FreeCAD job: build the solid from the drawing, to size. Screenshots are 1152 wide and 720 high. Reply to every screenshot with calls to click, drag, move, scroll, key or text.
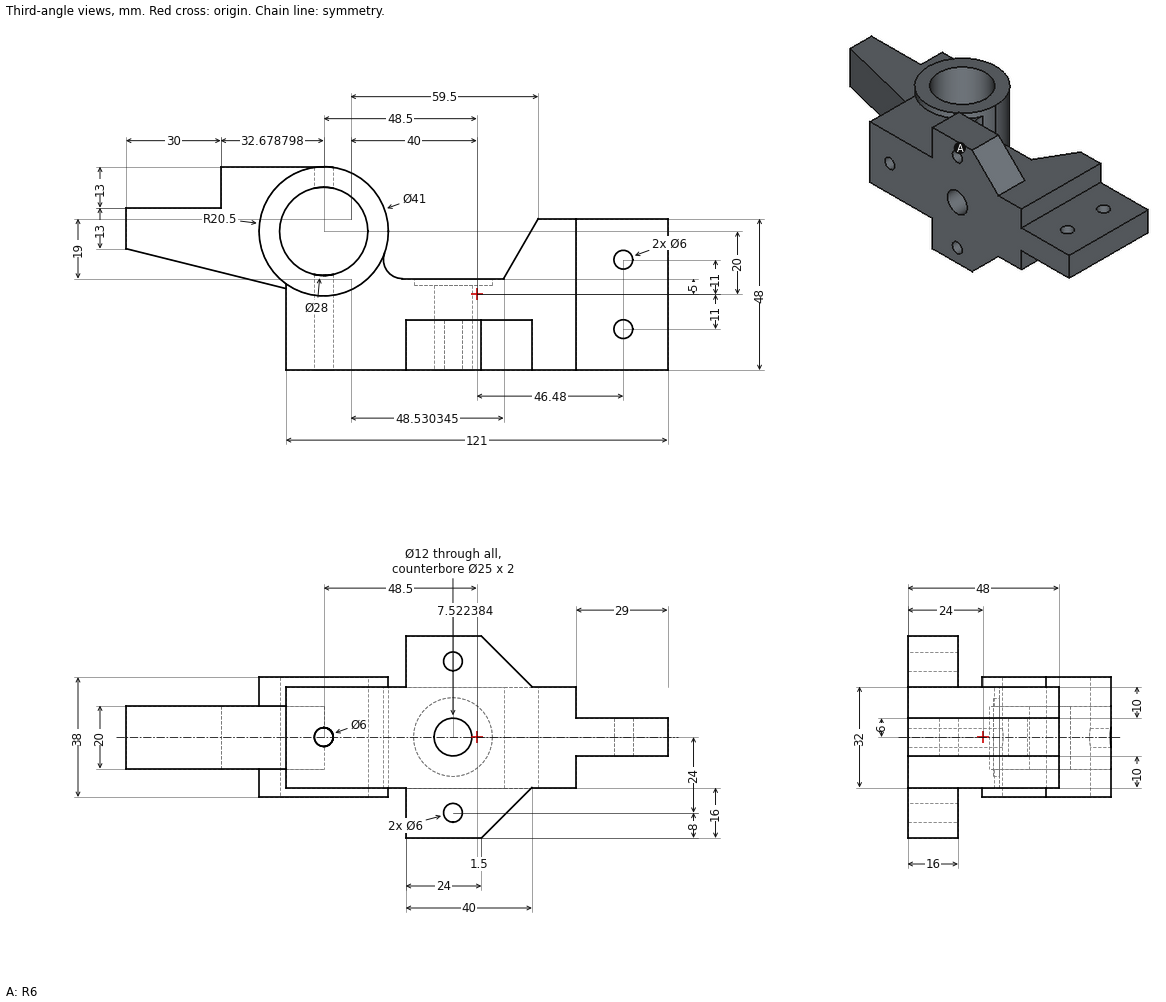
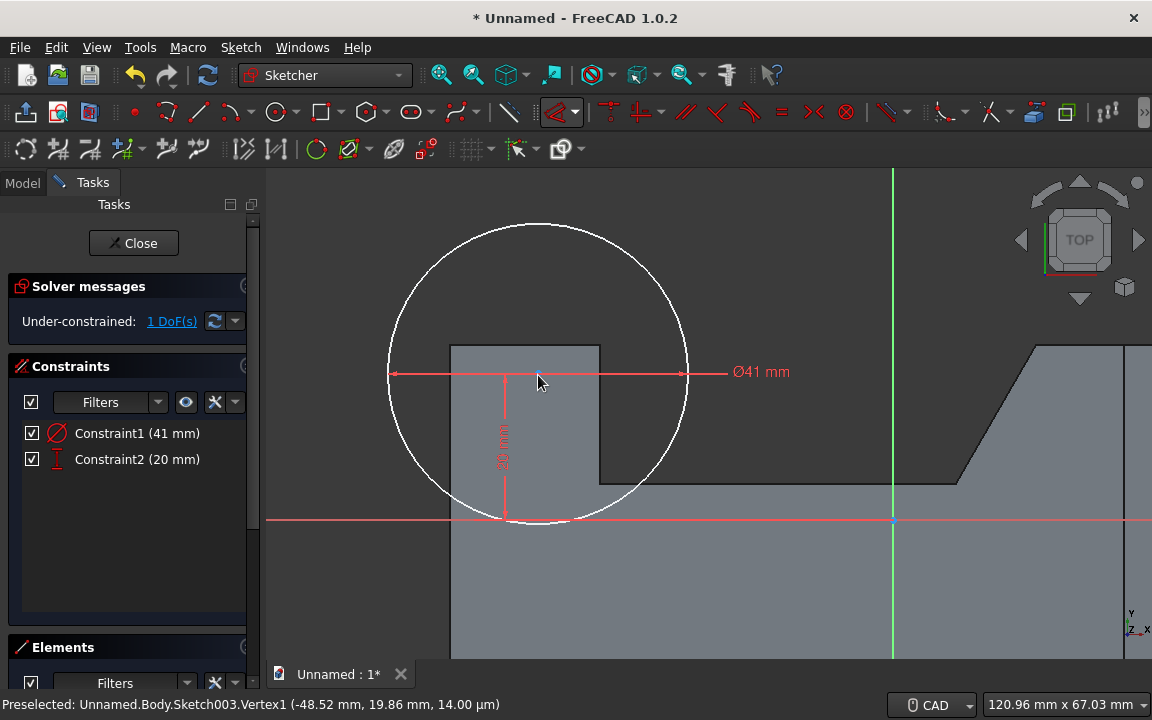
click(538, 374)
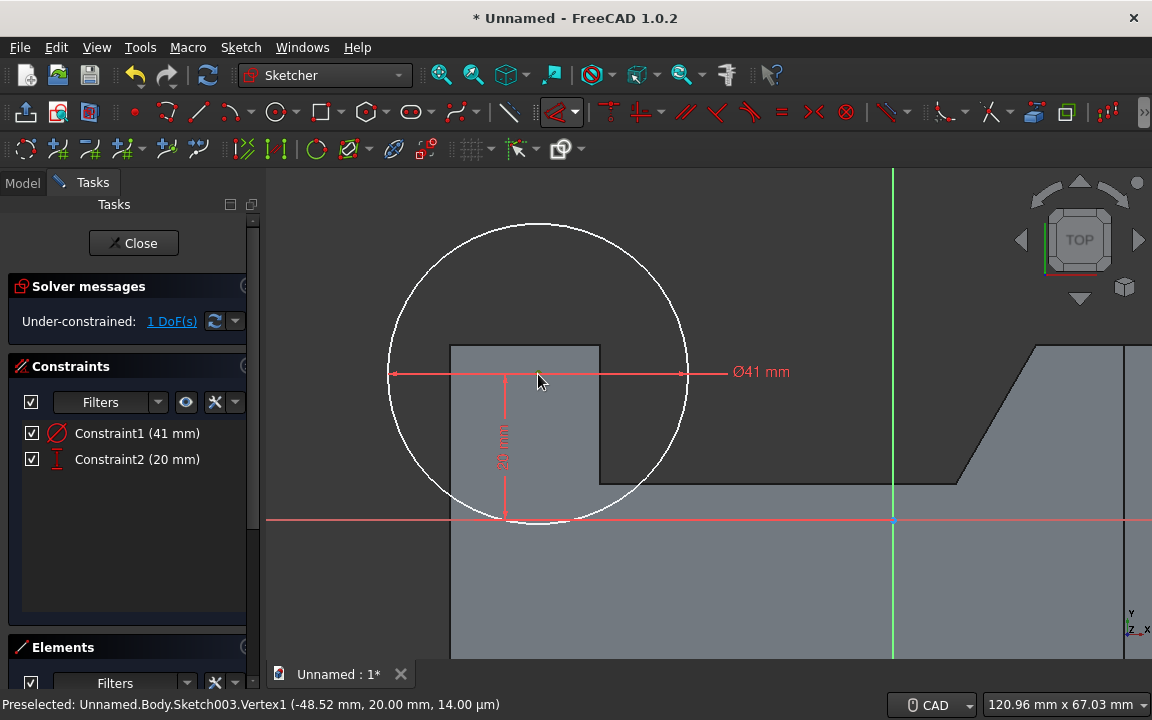
key(l)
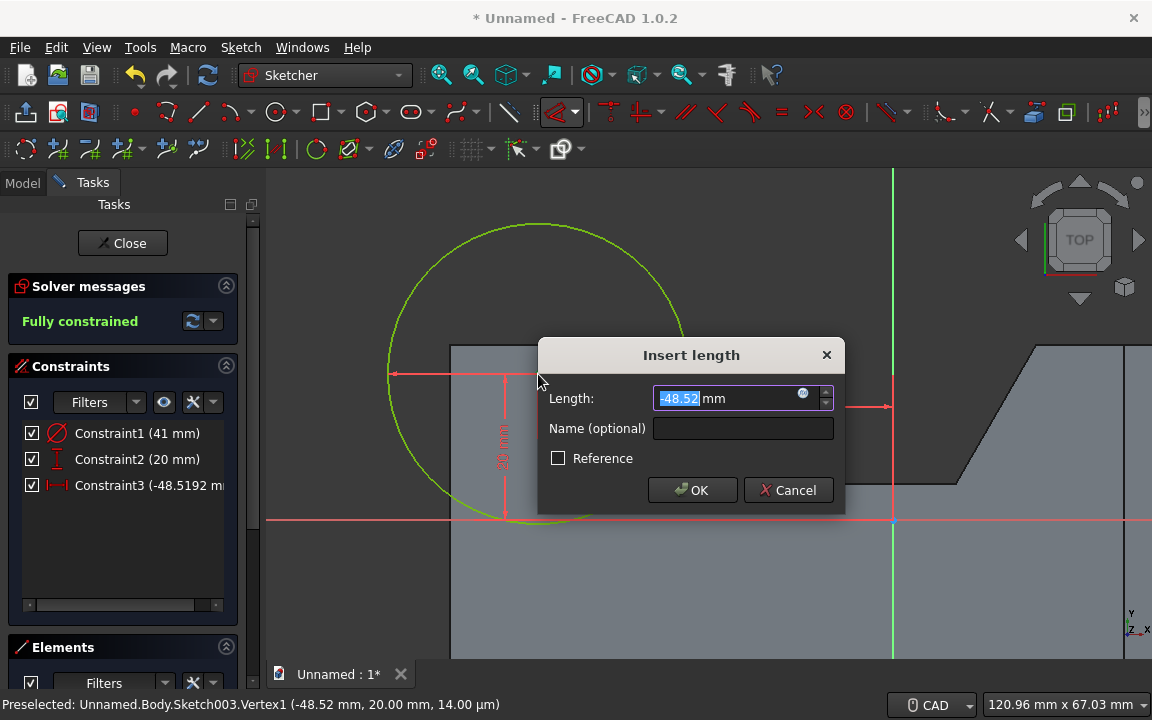
text(-48.5)
key(Return)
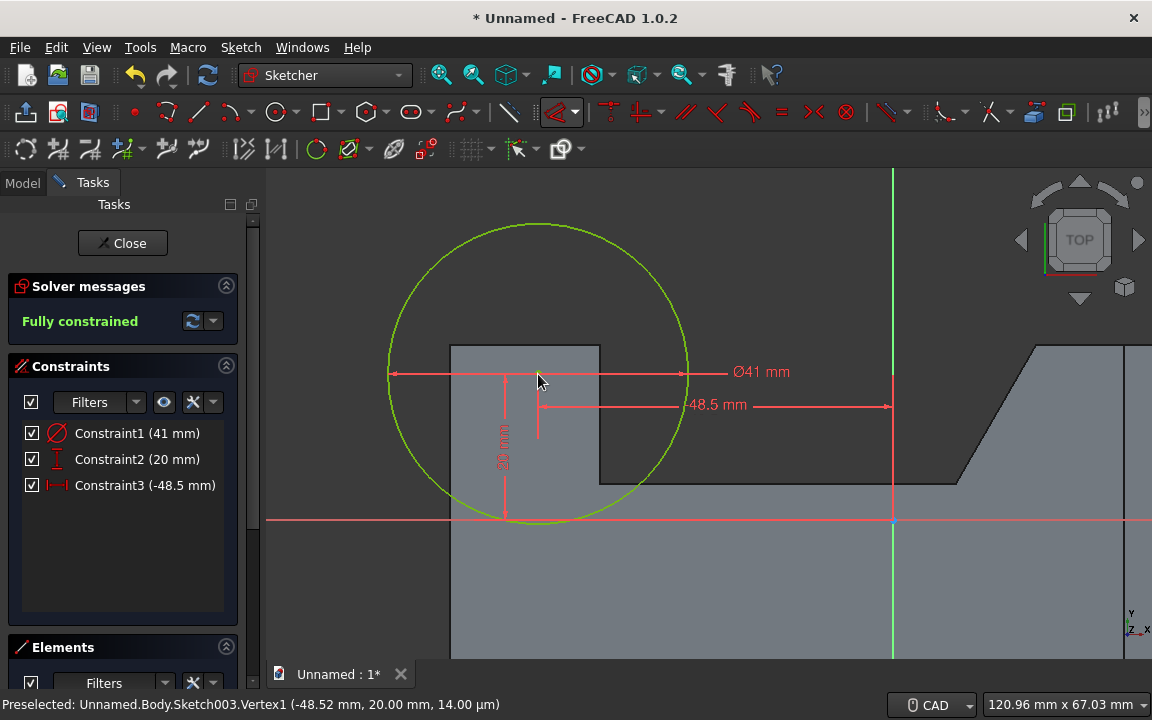
click(123, 243)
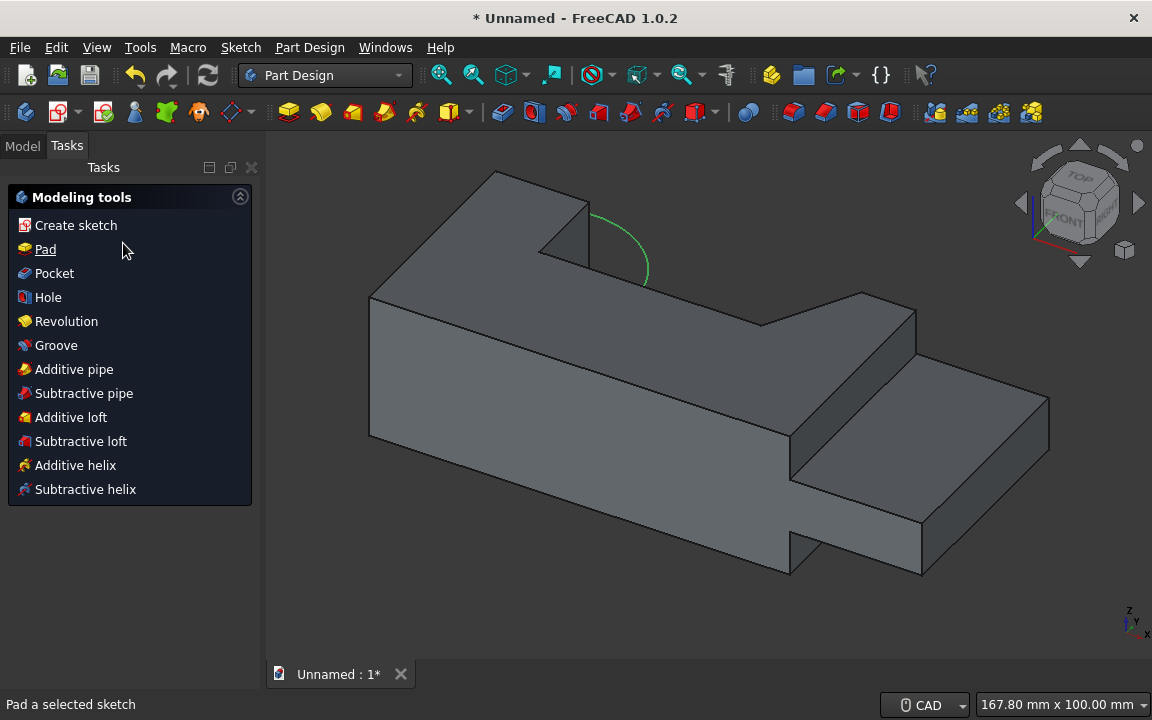
click(290, 112)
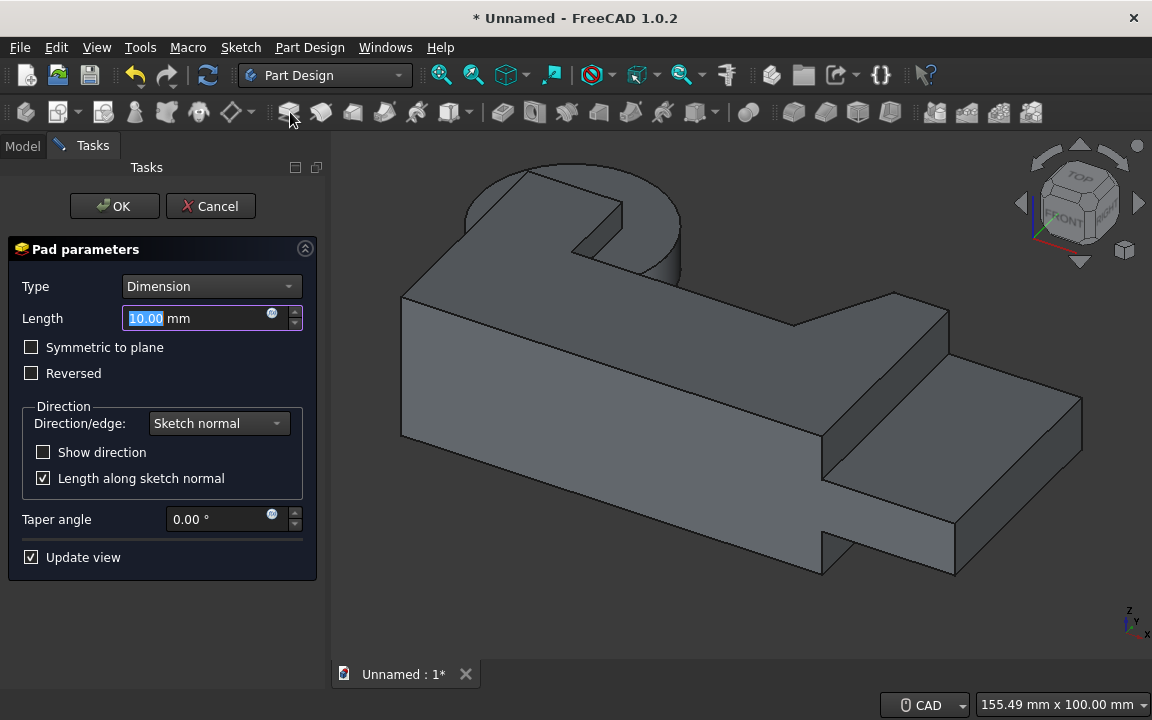
text(38)
key(Tab)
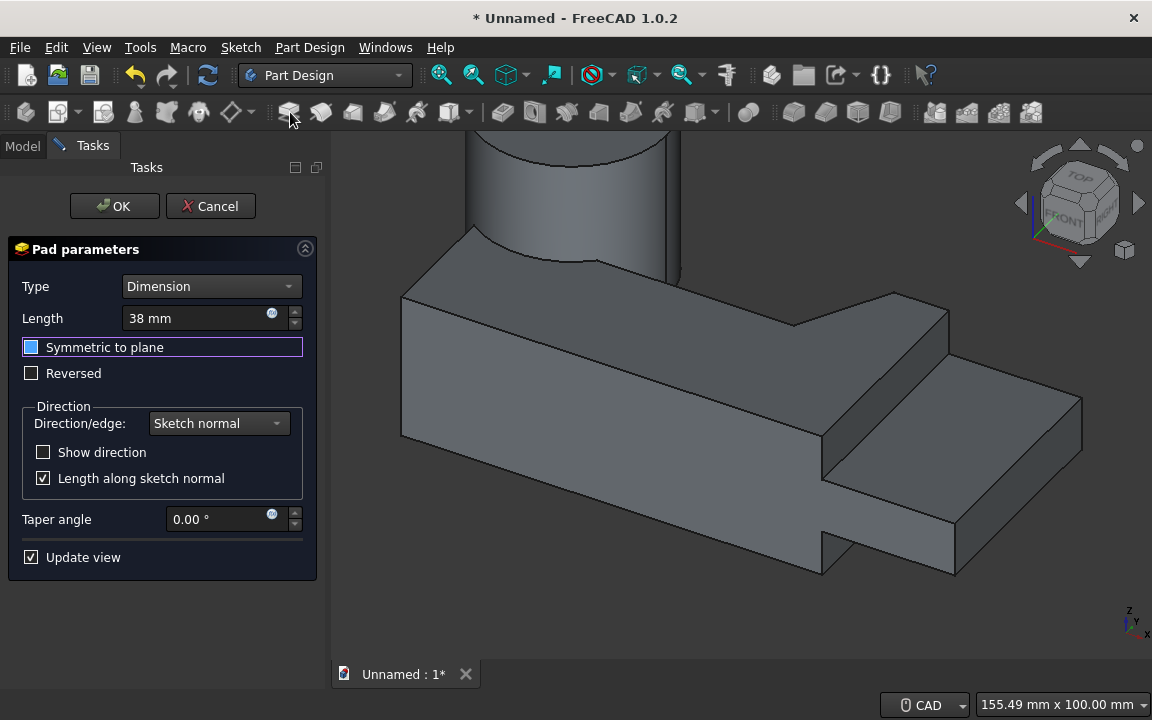
click(30, 347)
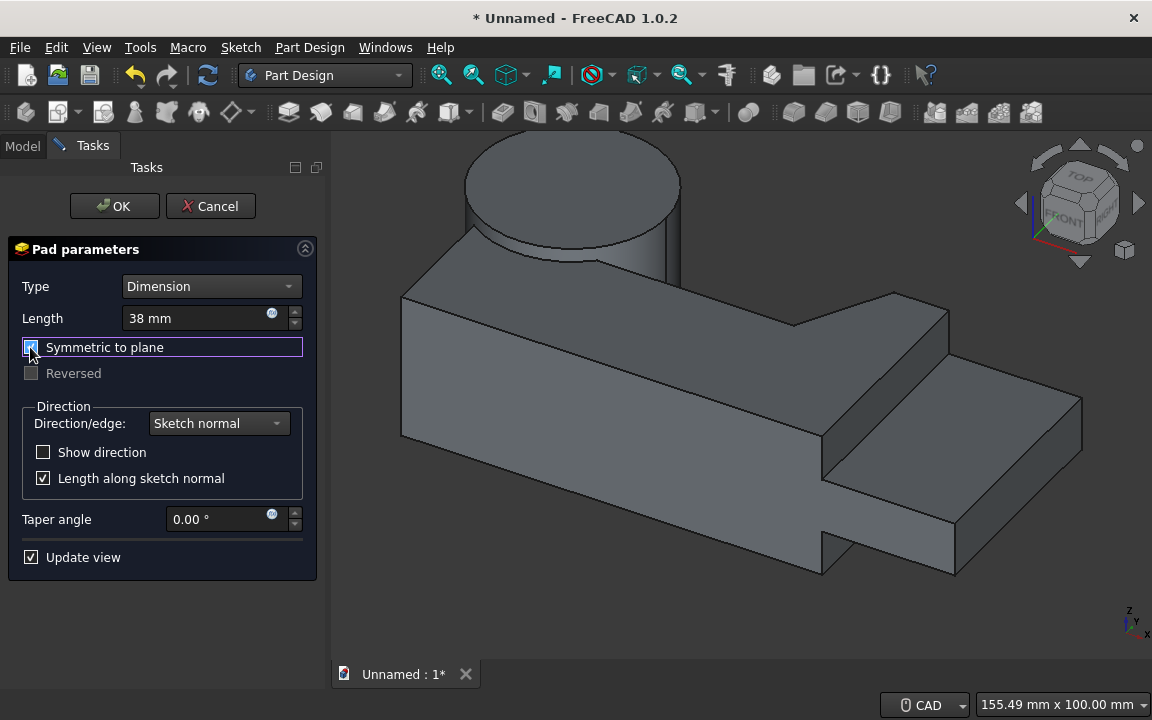
click(115, 206)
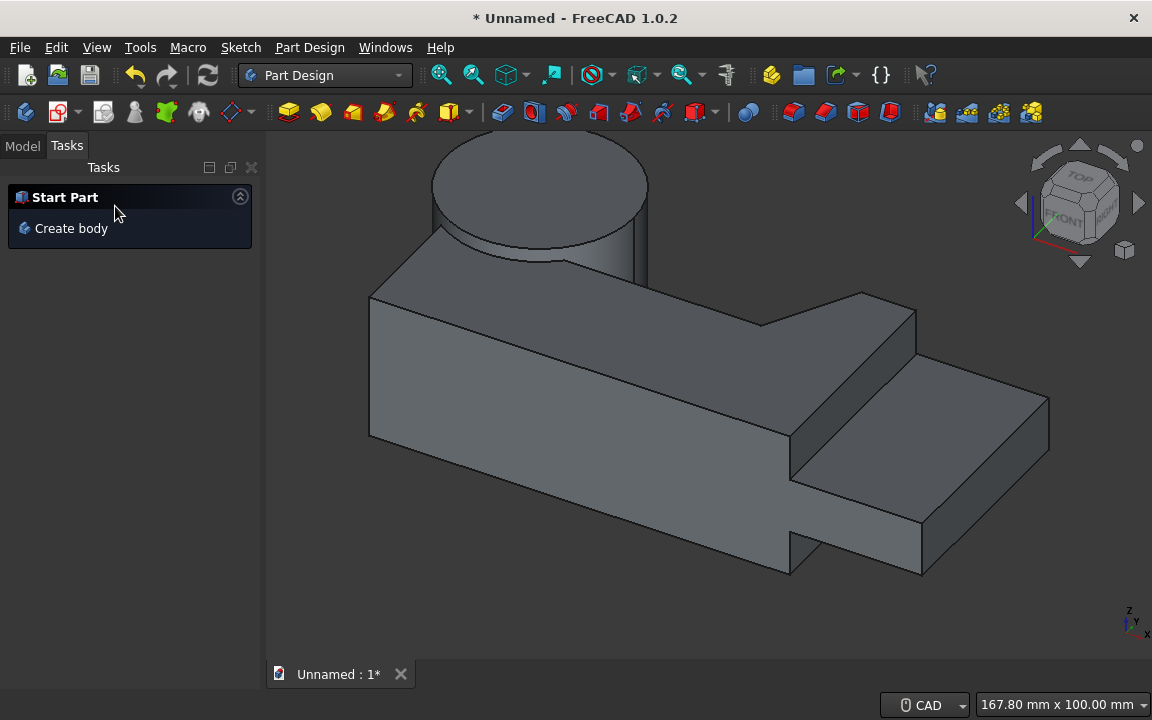
key(v)
key(f)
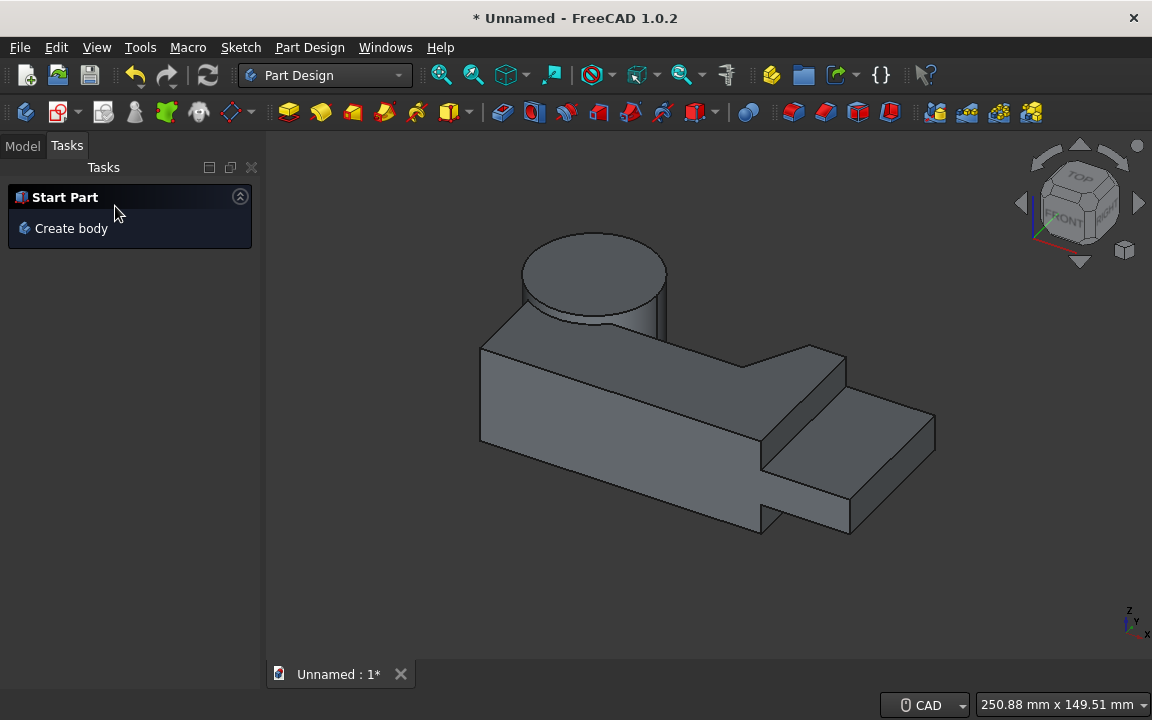
key(0)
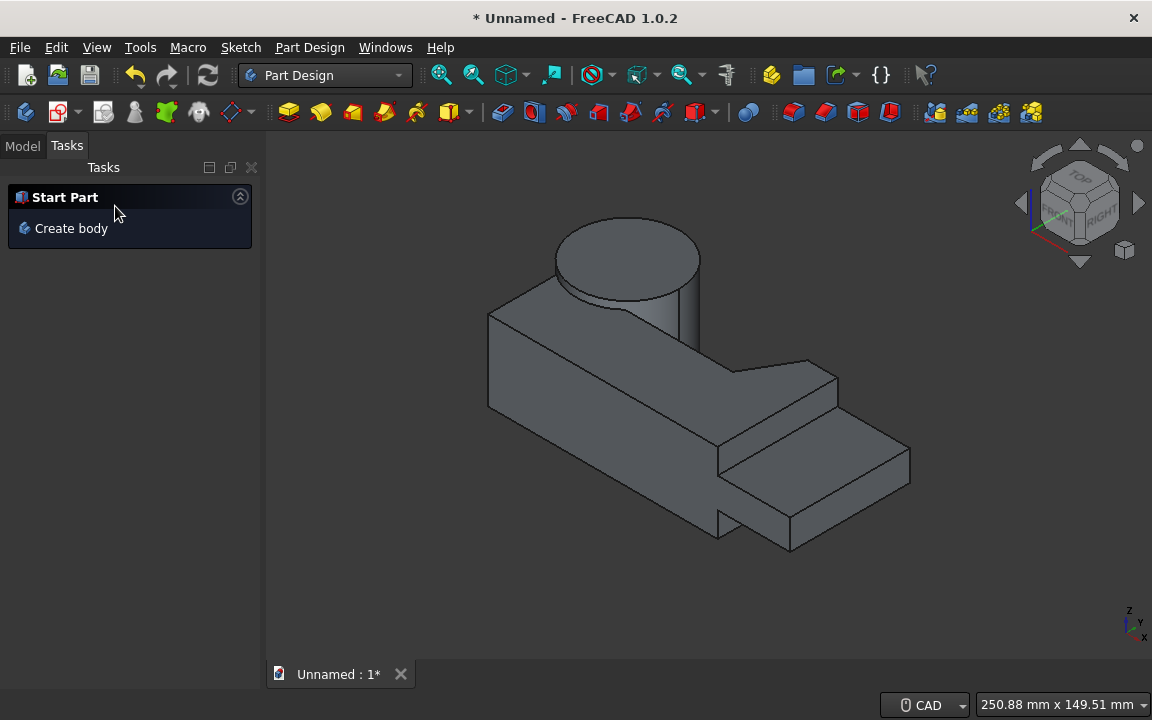
key(2)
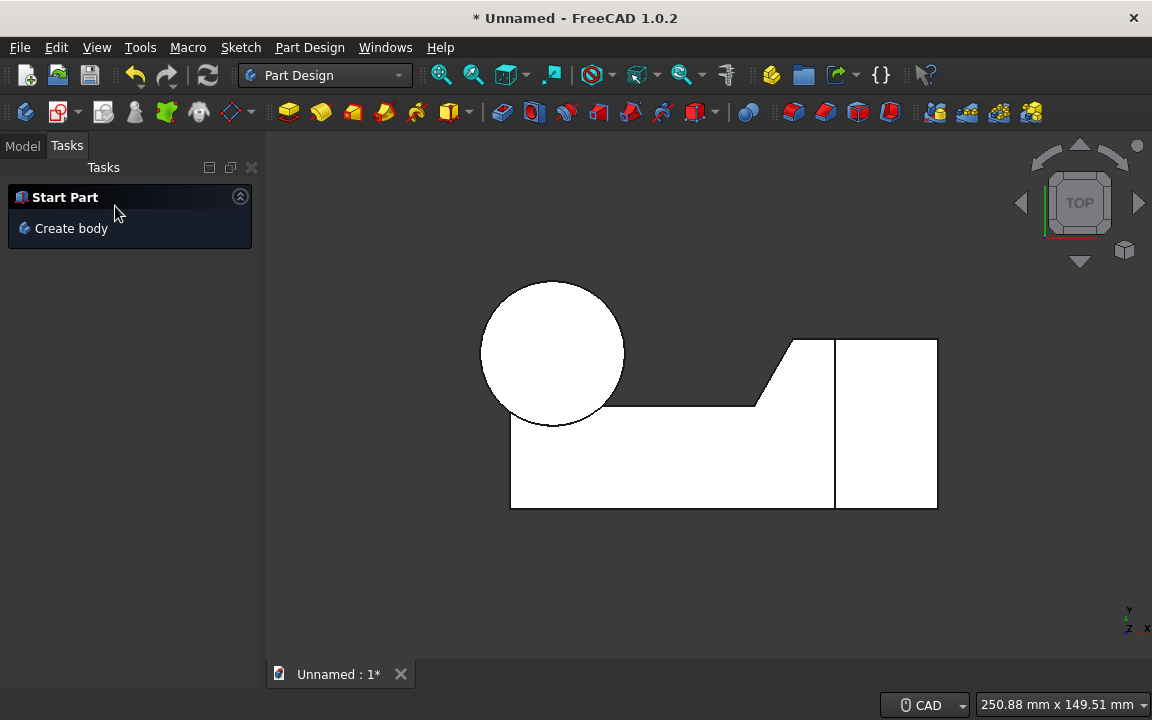
key(1)